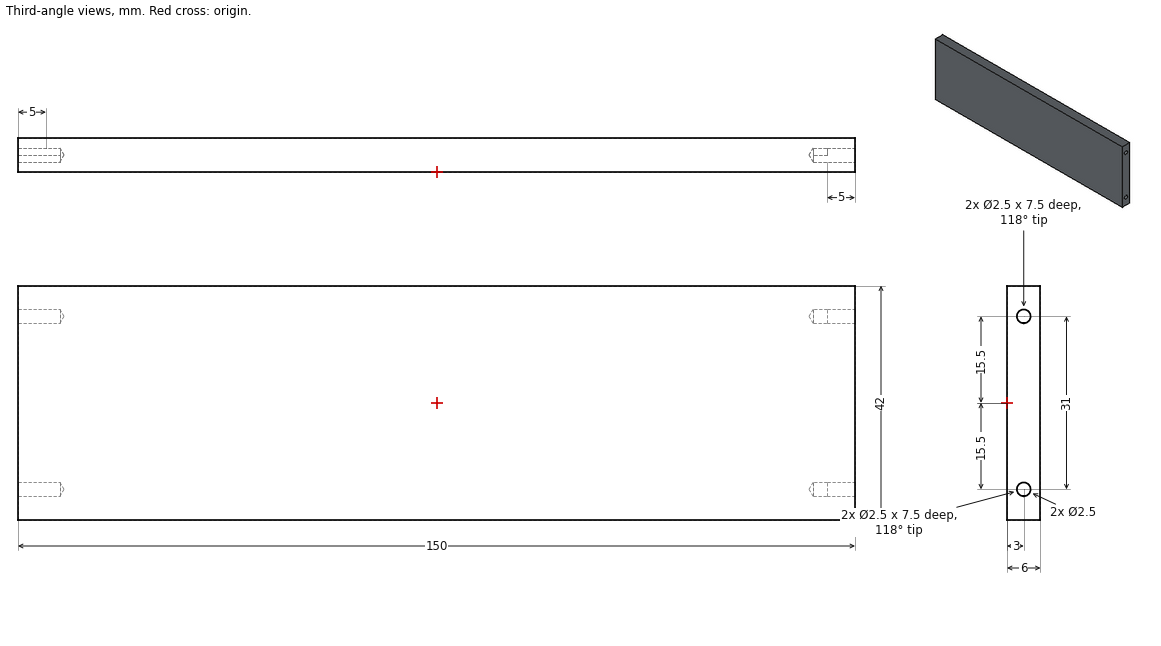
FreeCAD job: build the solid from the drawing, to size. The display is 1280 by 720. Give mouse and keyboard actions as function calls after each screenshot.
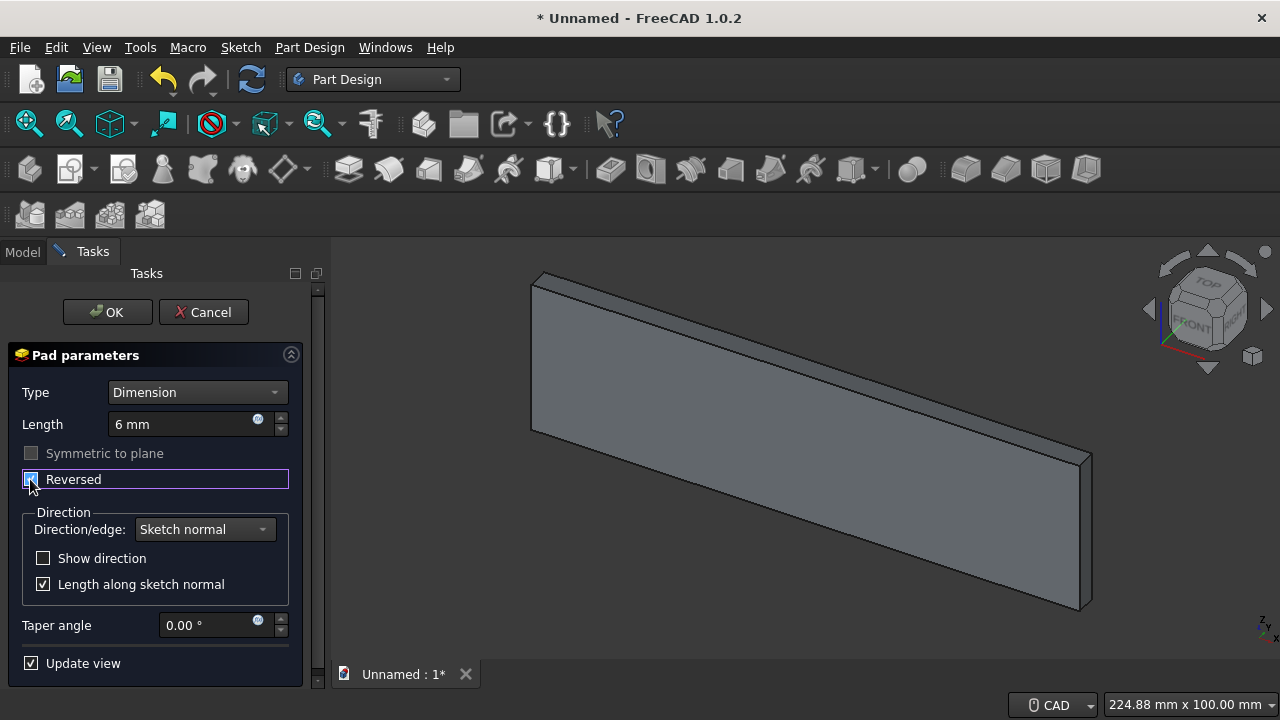
click(108, 312)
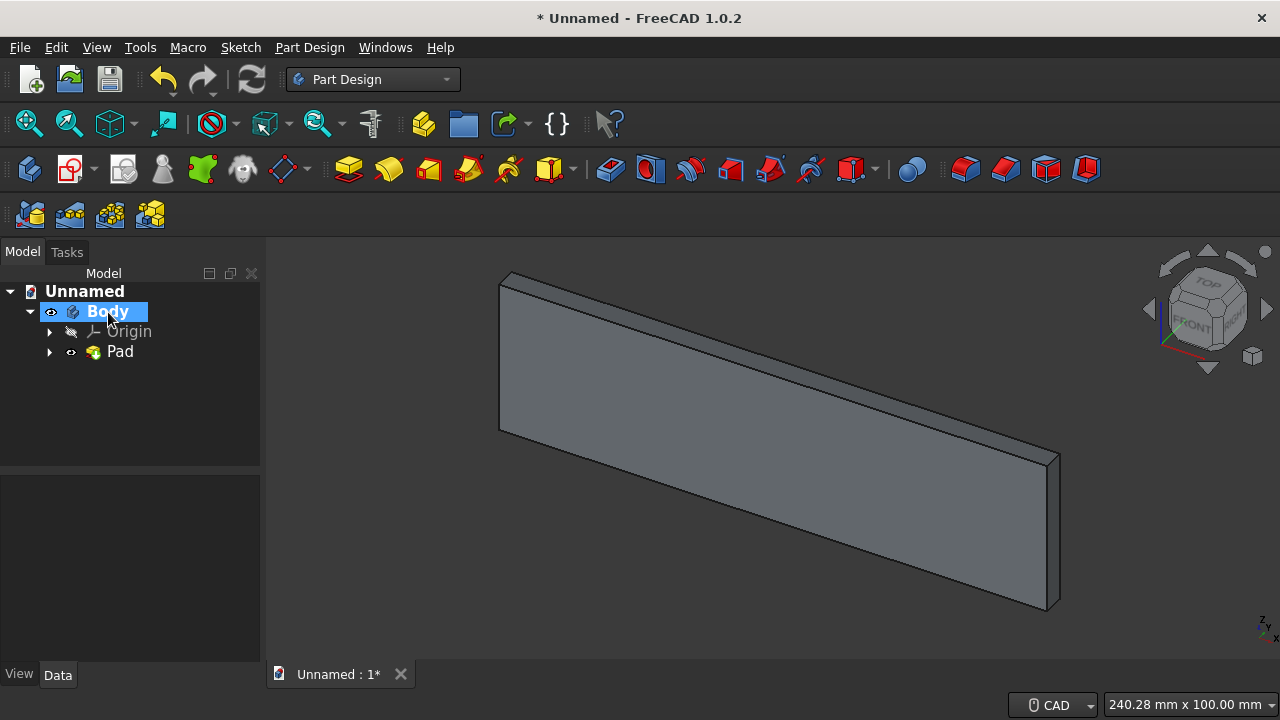
key(0)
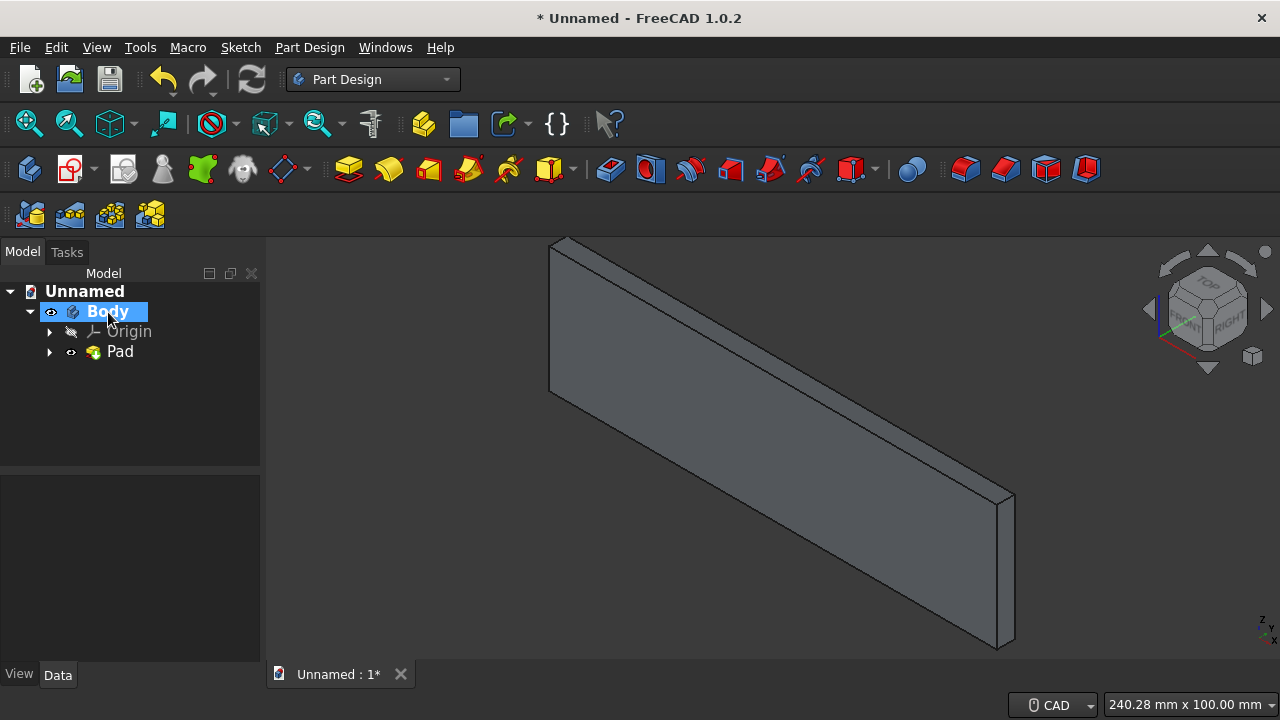
click(30, 124)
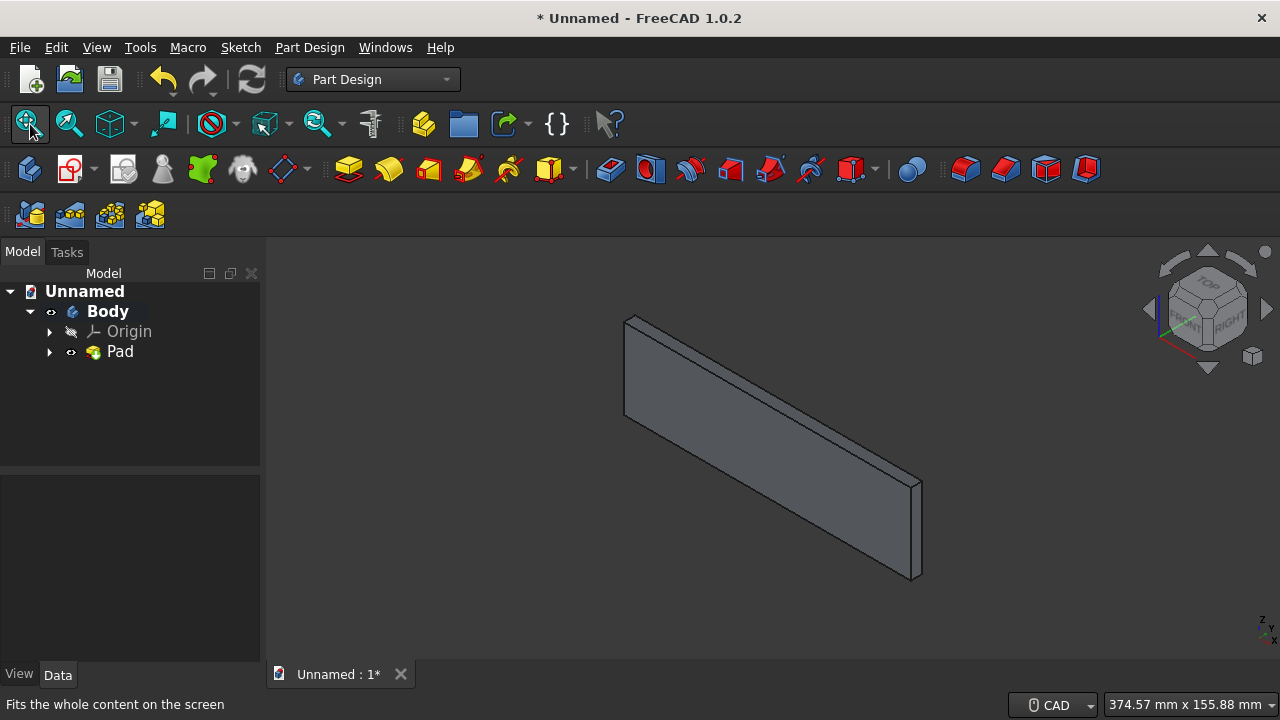
key(3)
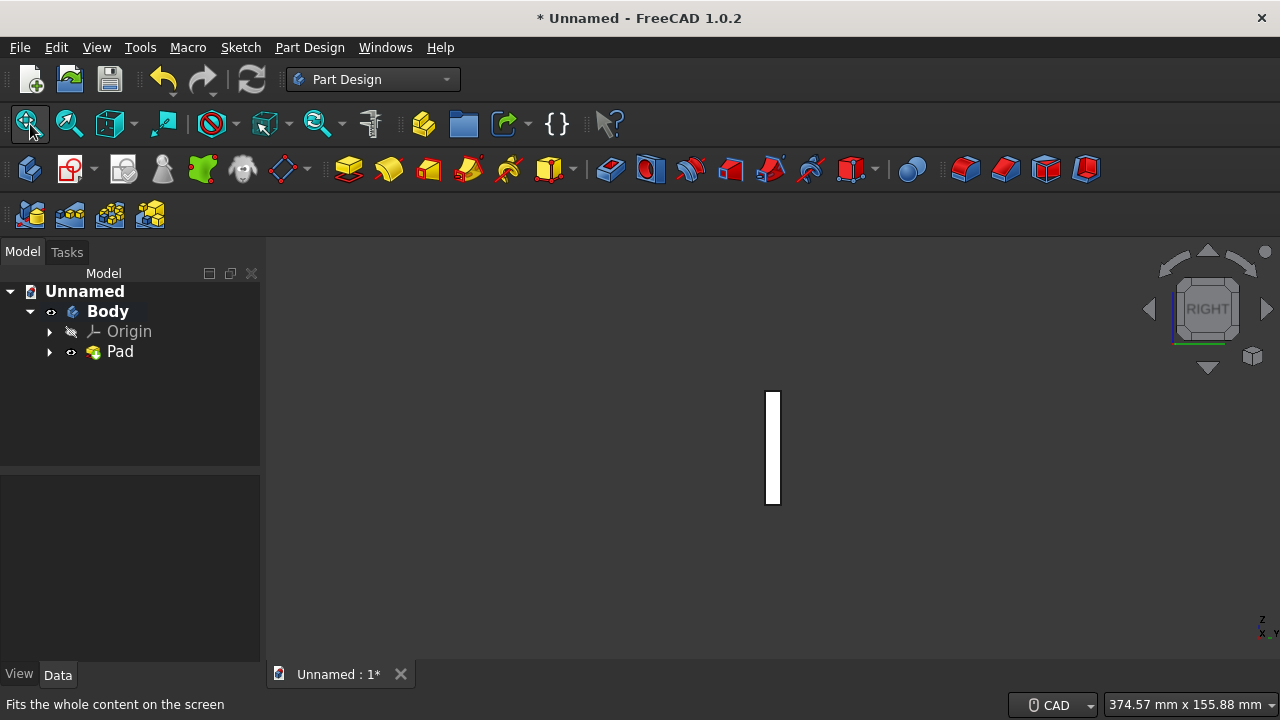
click(30, 124)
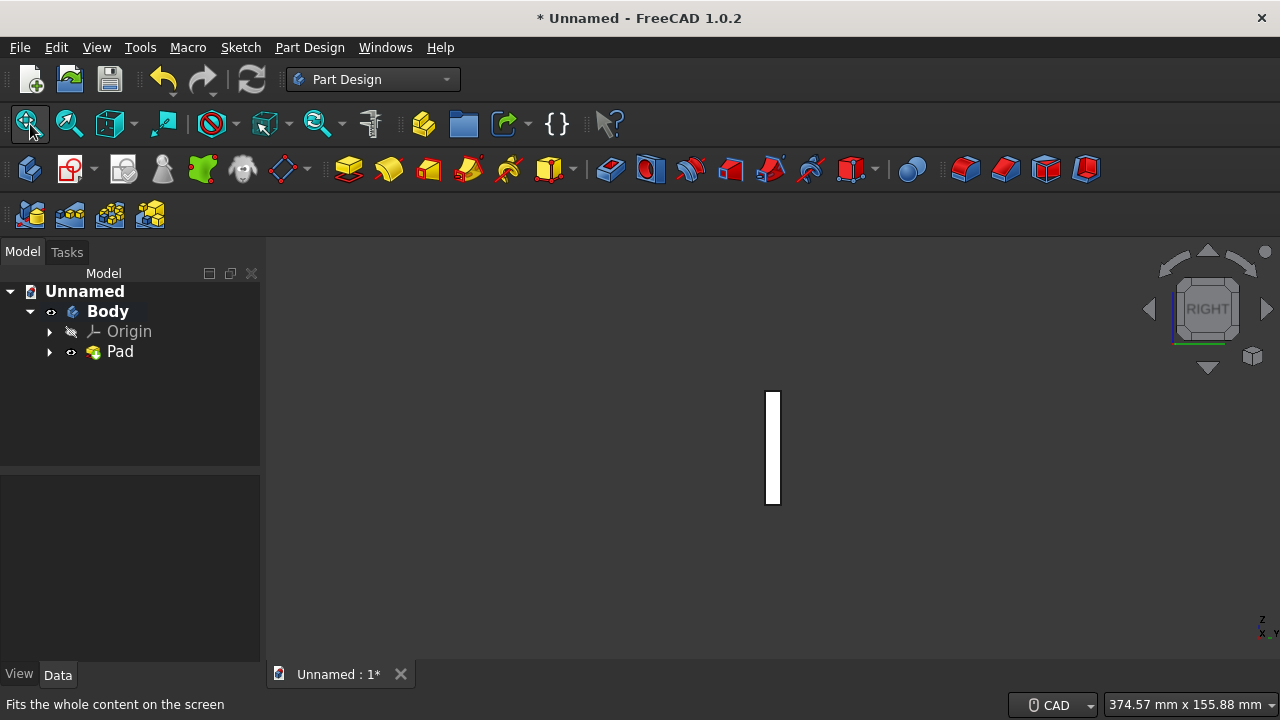
click(773, 415)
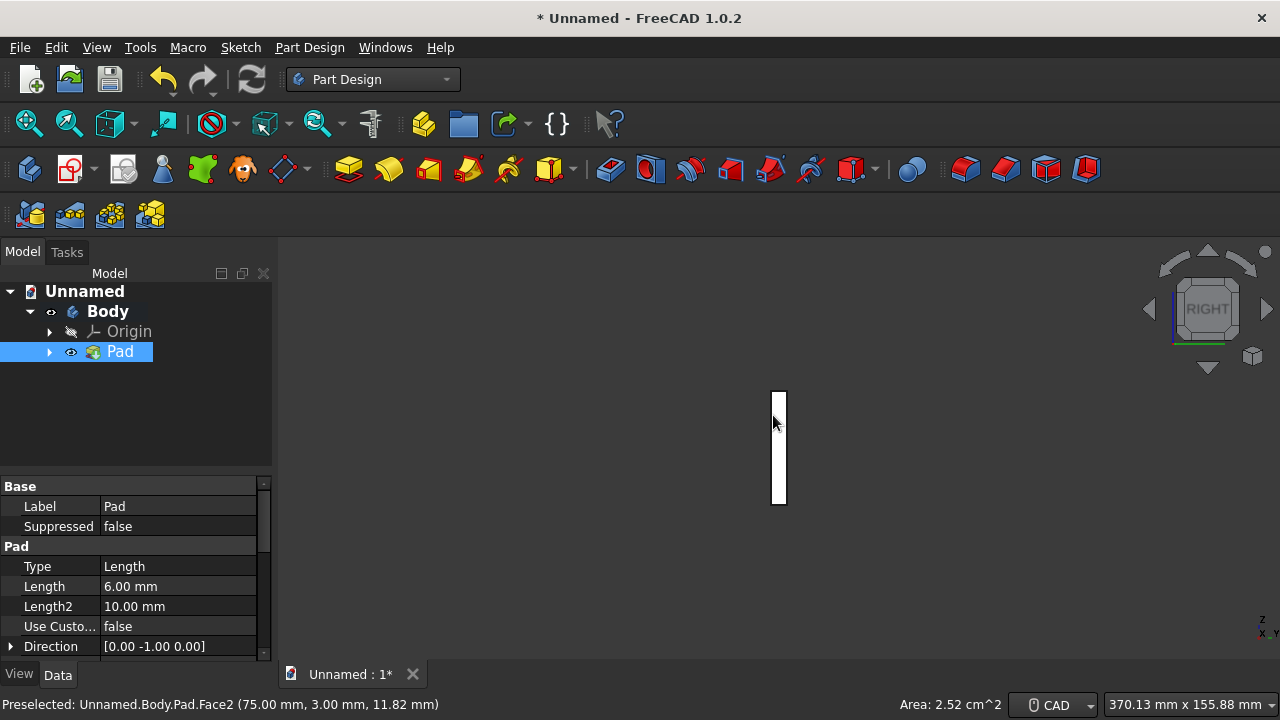
click(70, 170)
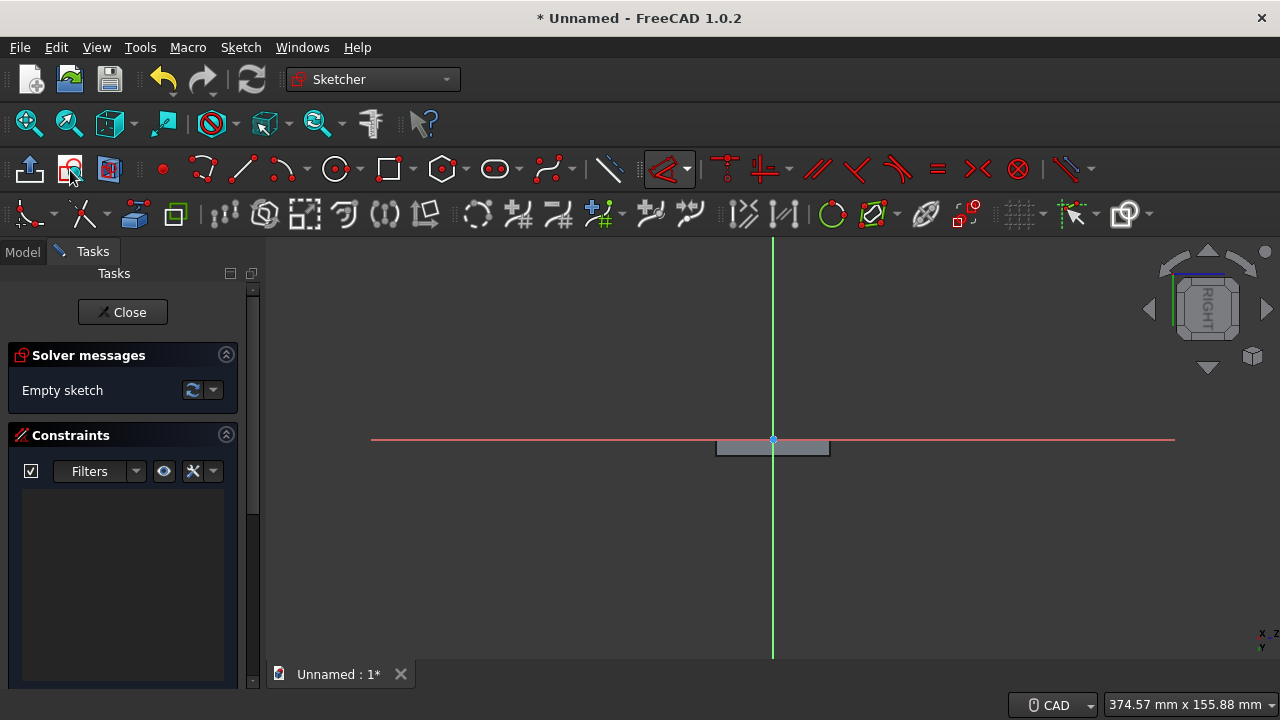
scroll(787, 445, up, 9)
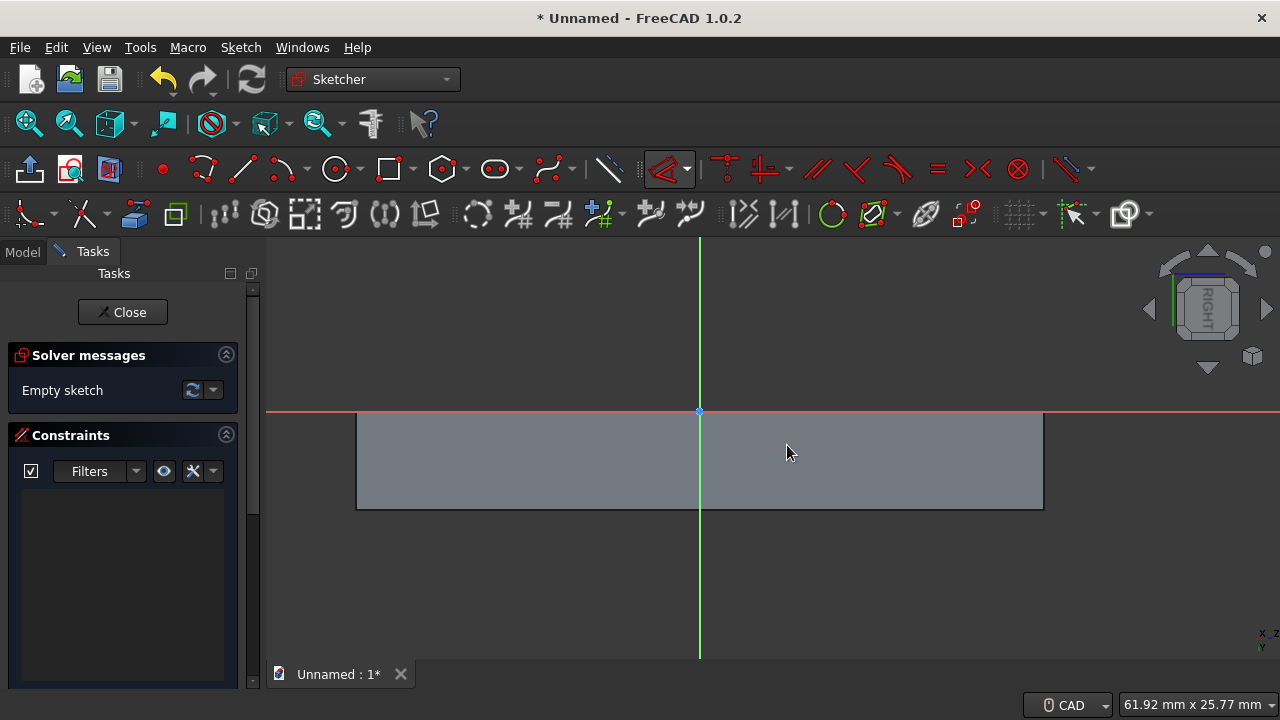
click(336, 170)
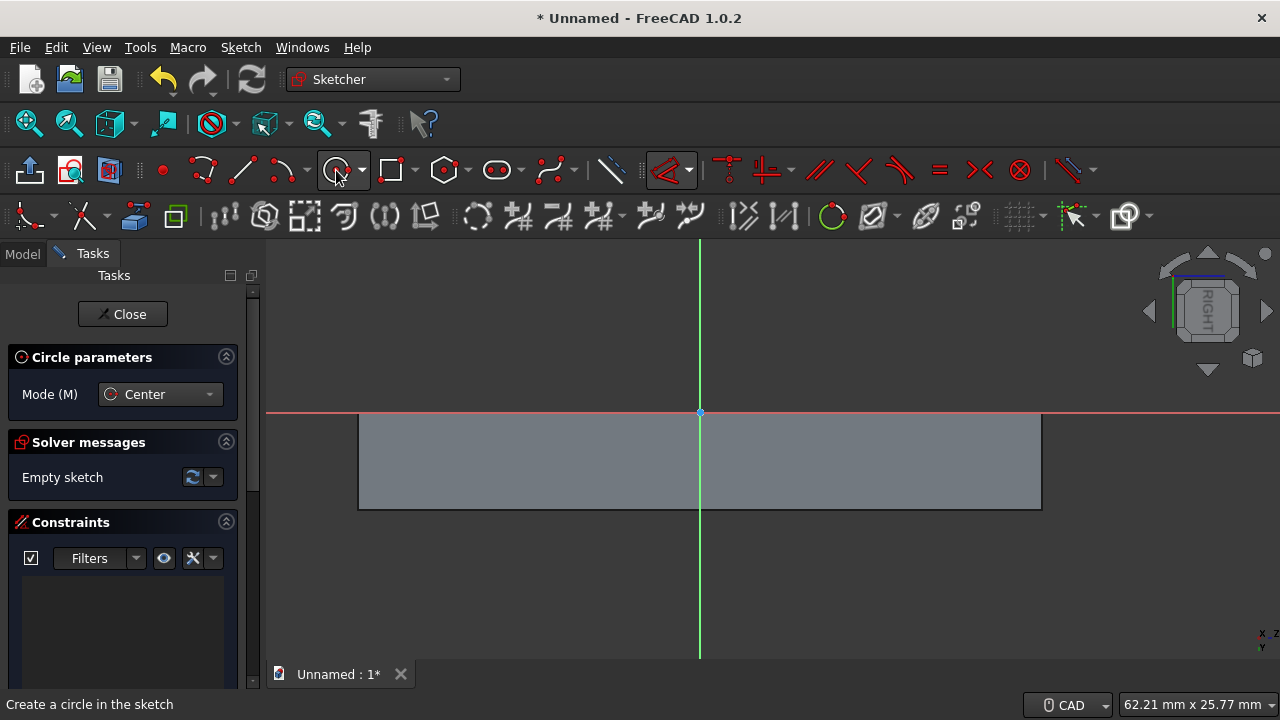
click(447, 462)
move(462, 447)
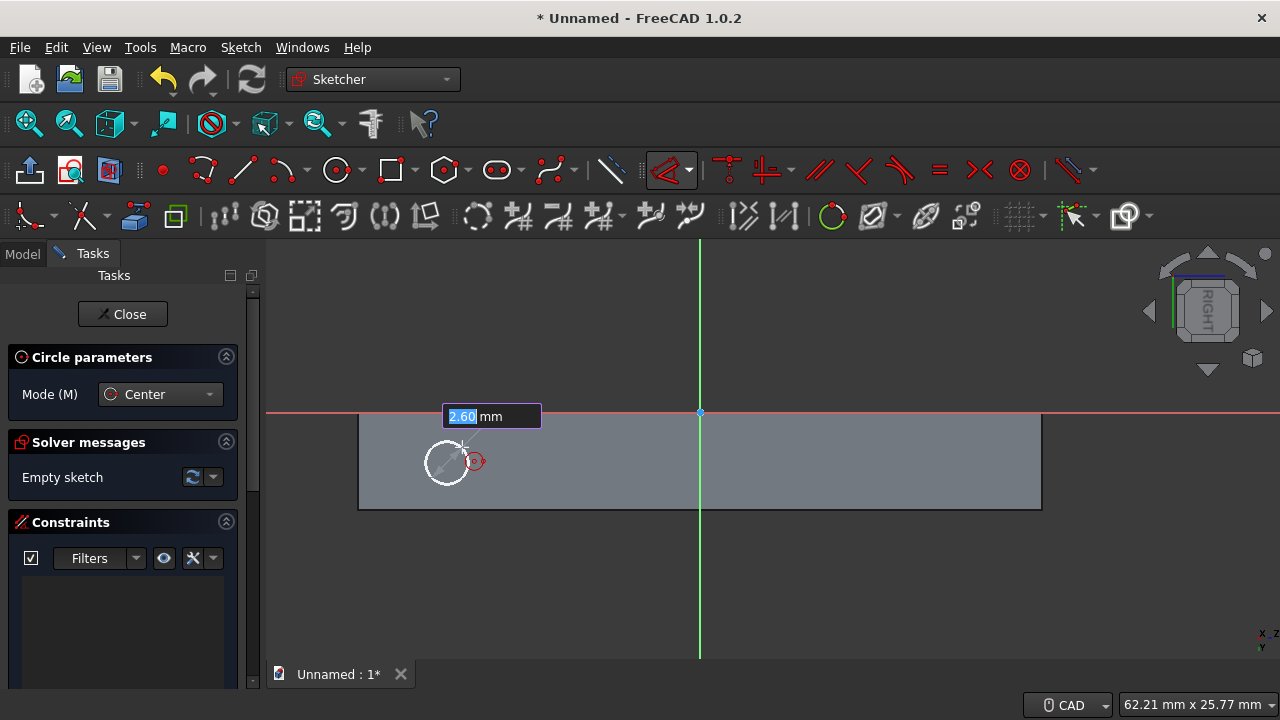
text(2.5)
key(Return)